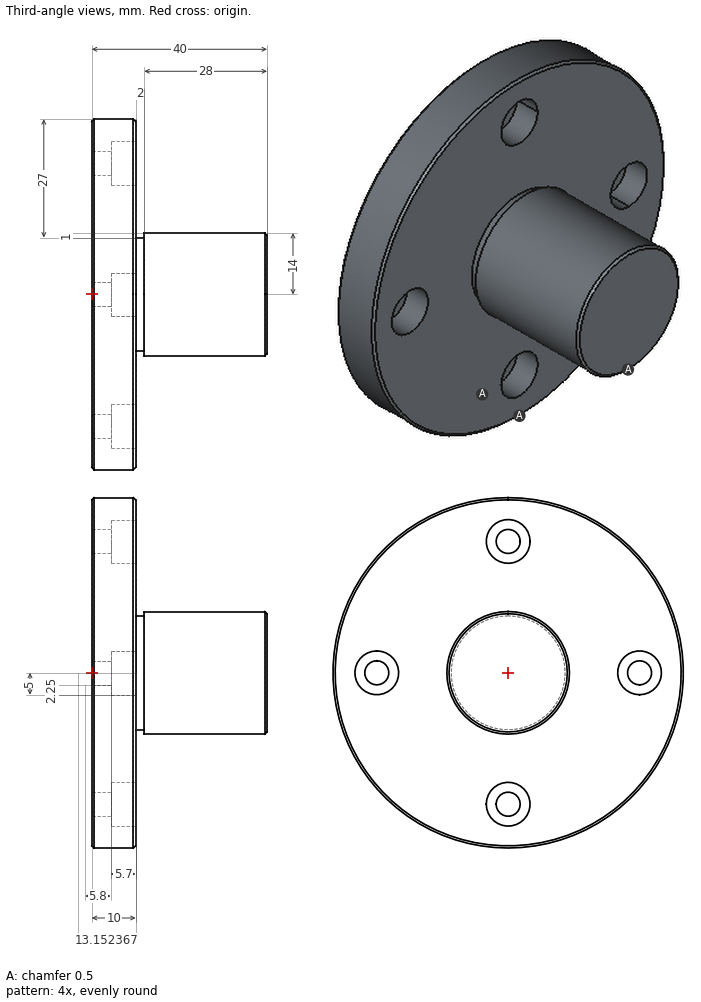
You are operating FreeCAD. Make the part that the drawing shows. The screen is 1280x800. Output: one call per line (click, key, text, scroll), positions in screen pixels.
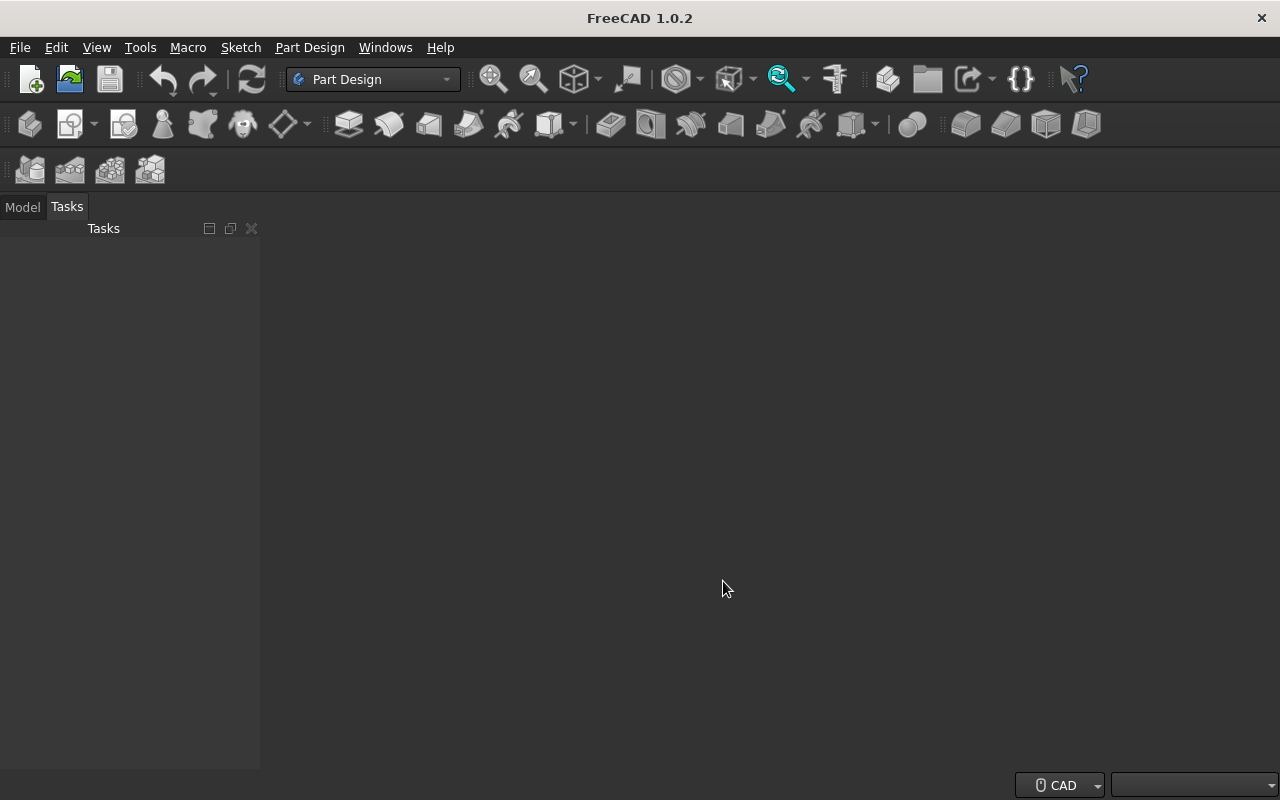
click(30, 80)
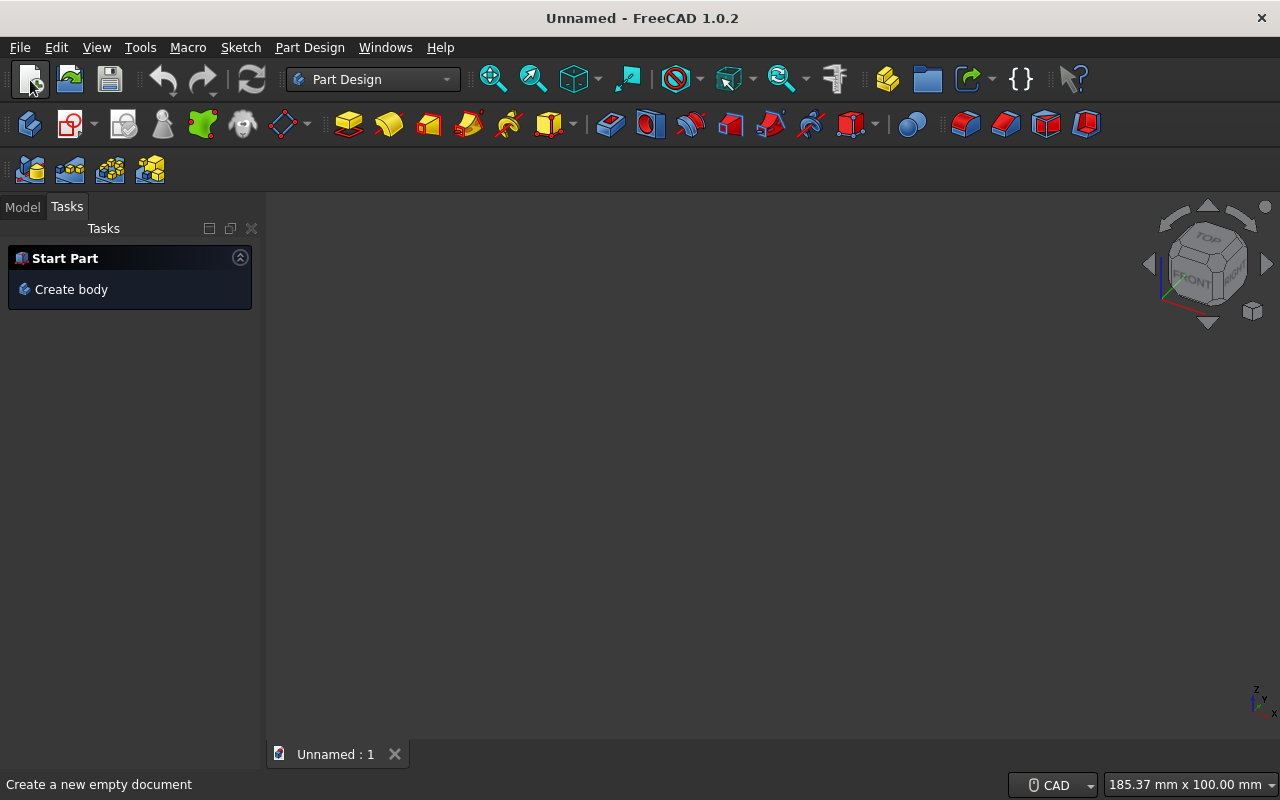
click(70, 124)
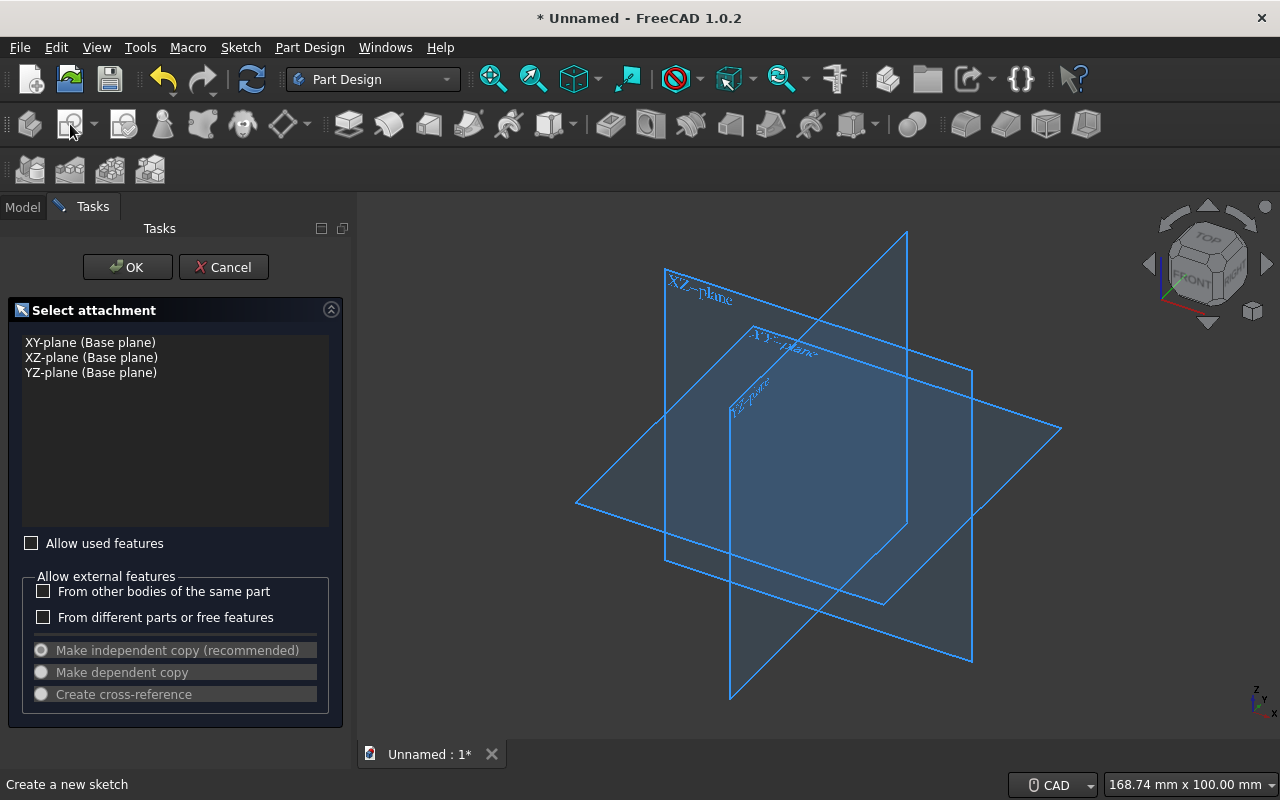
click(82, 342)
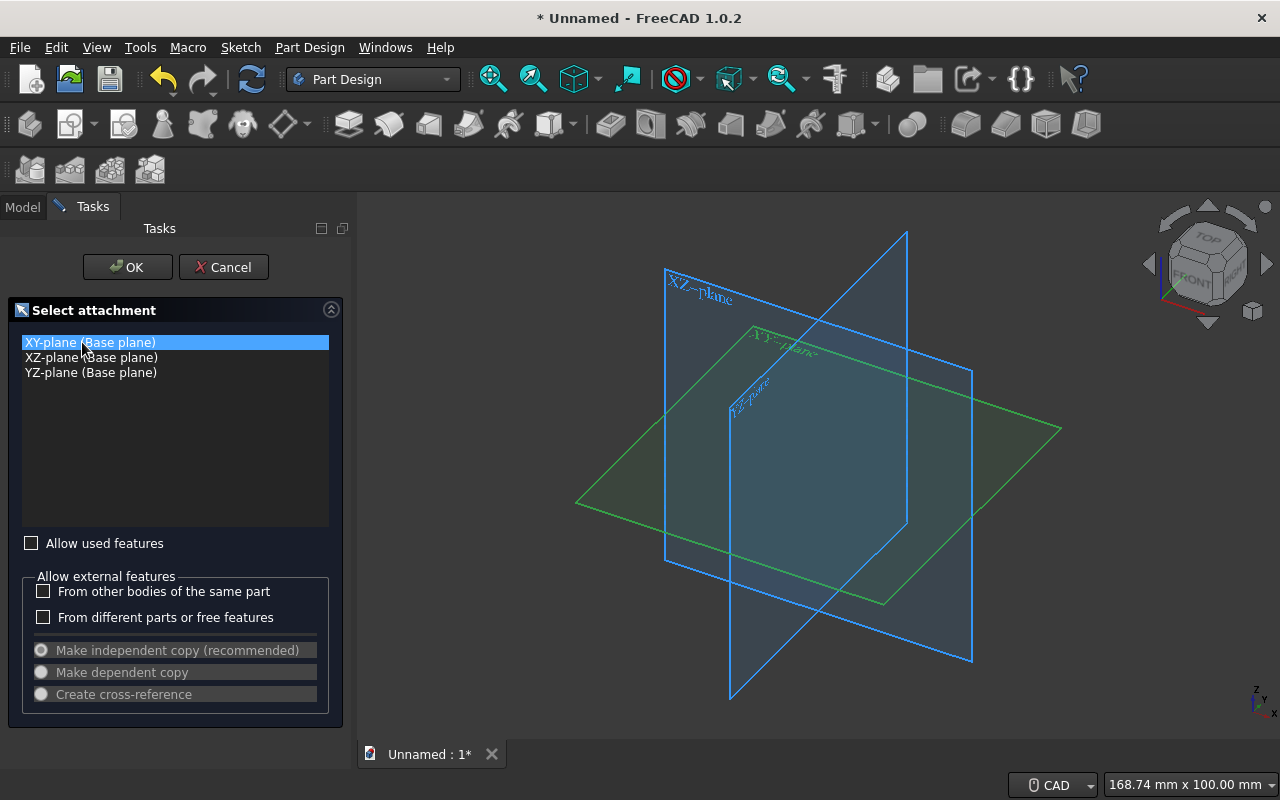
click(128, 267)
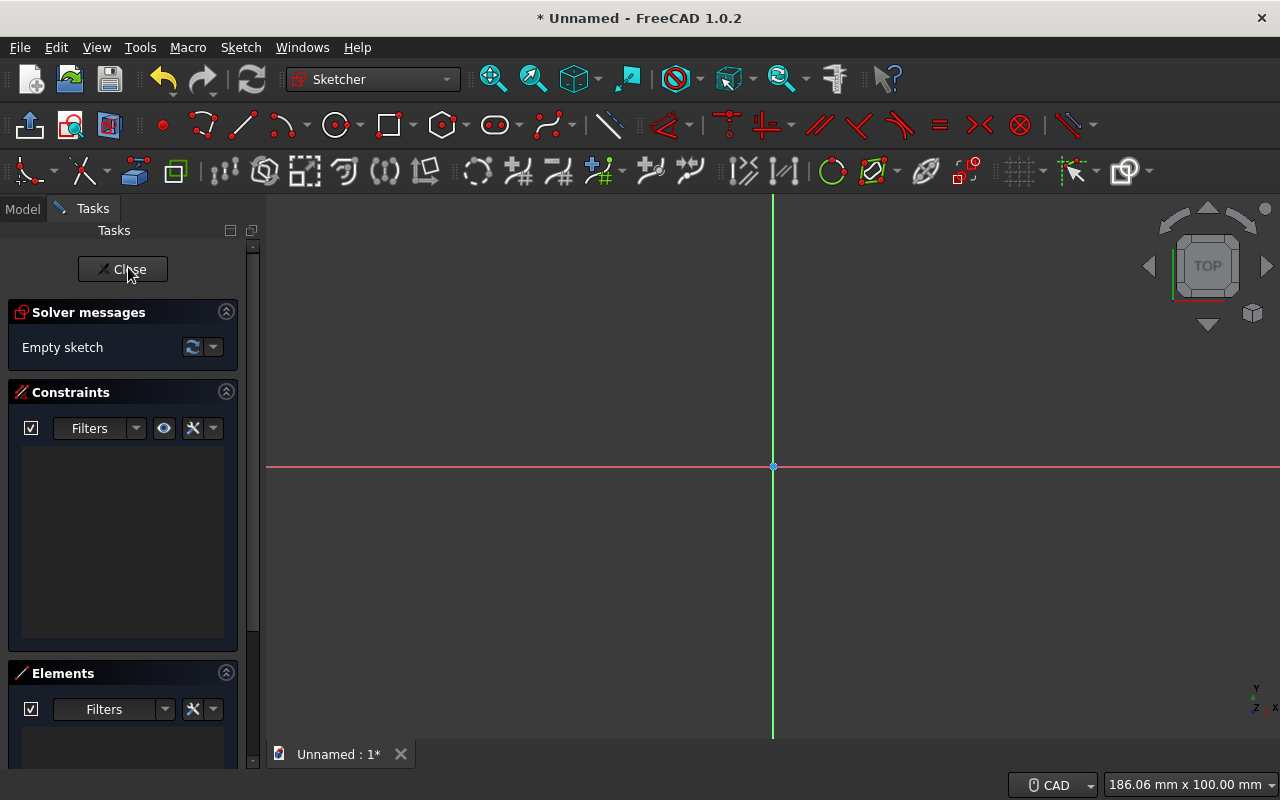
scroll(1115, 222, up, 2)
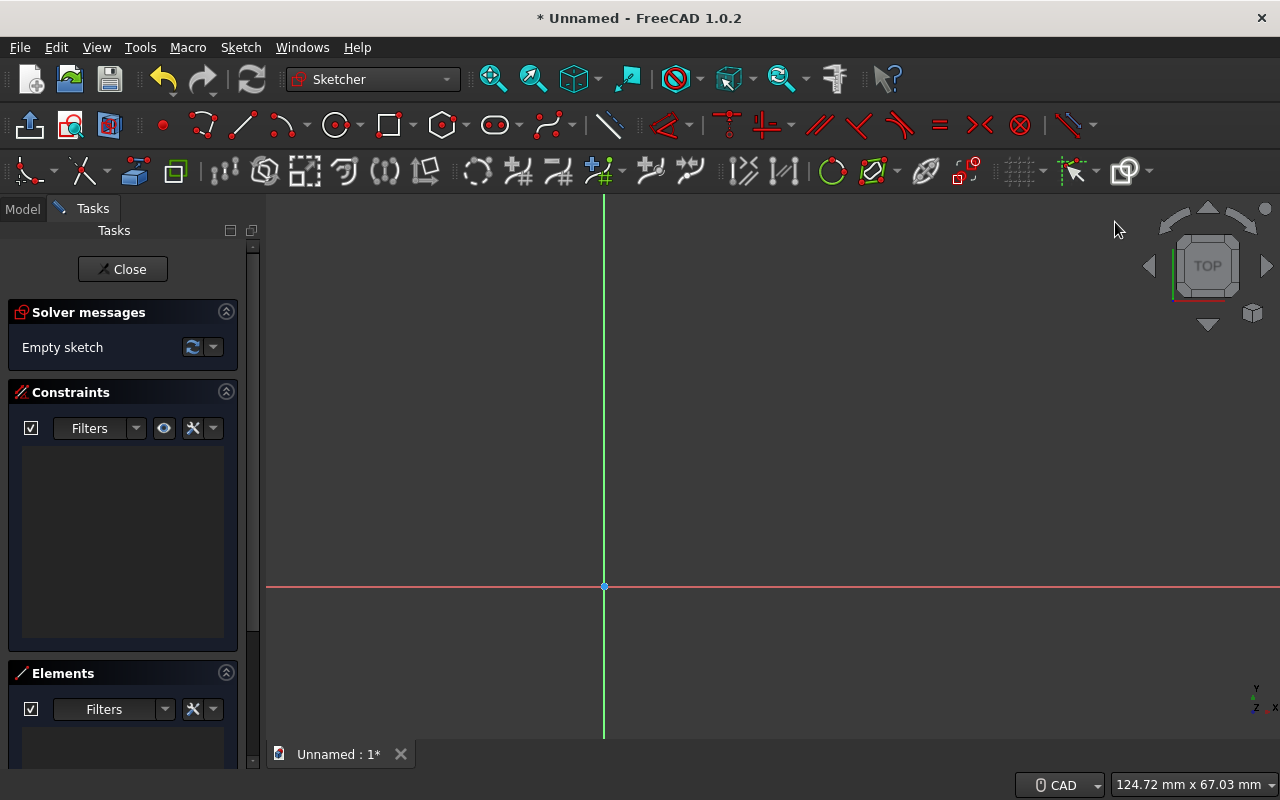
click(204, 126)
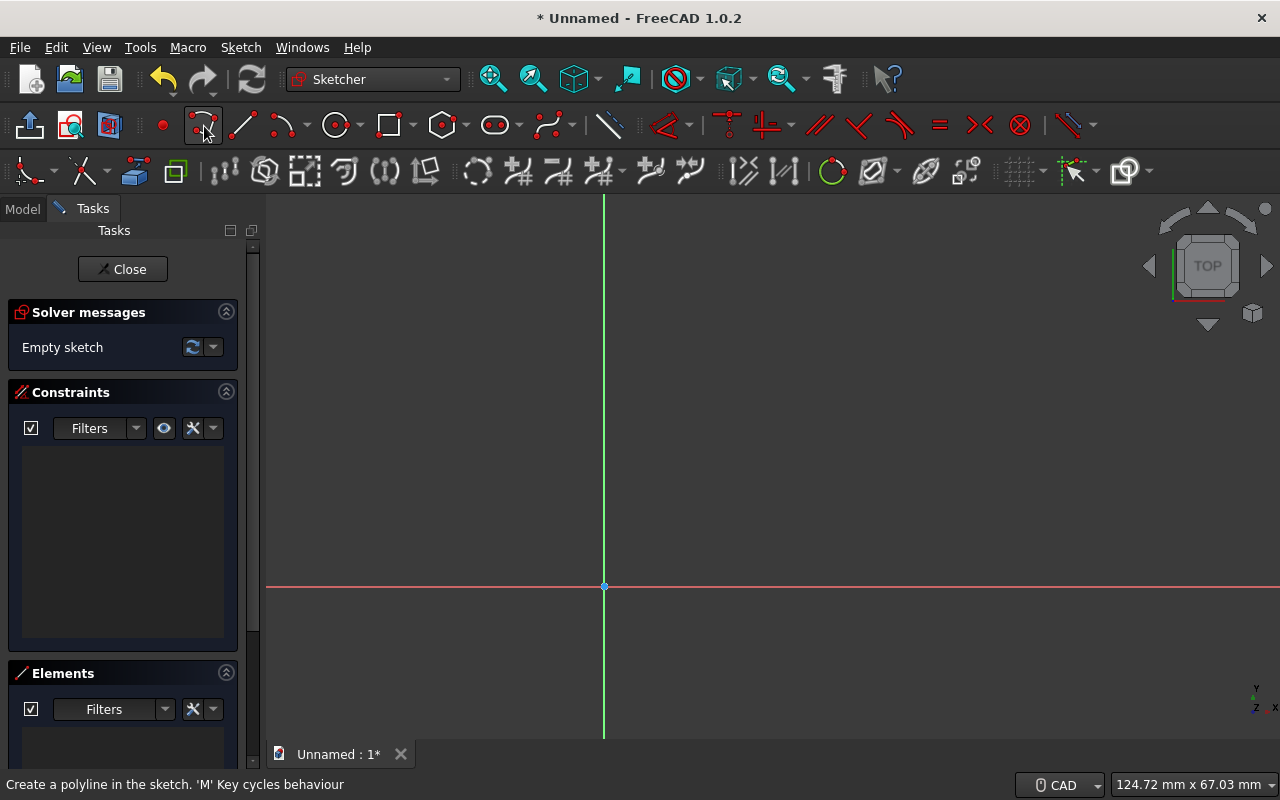
click(604, 587)
click(930, 578)
click(930, 473)
click(702, 473)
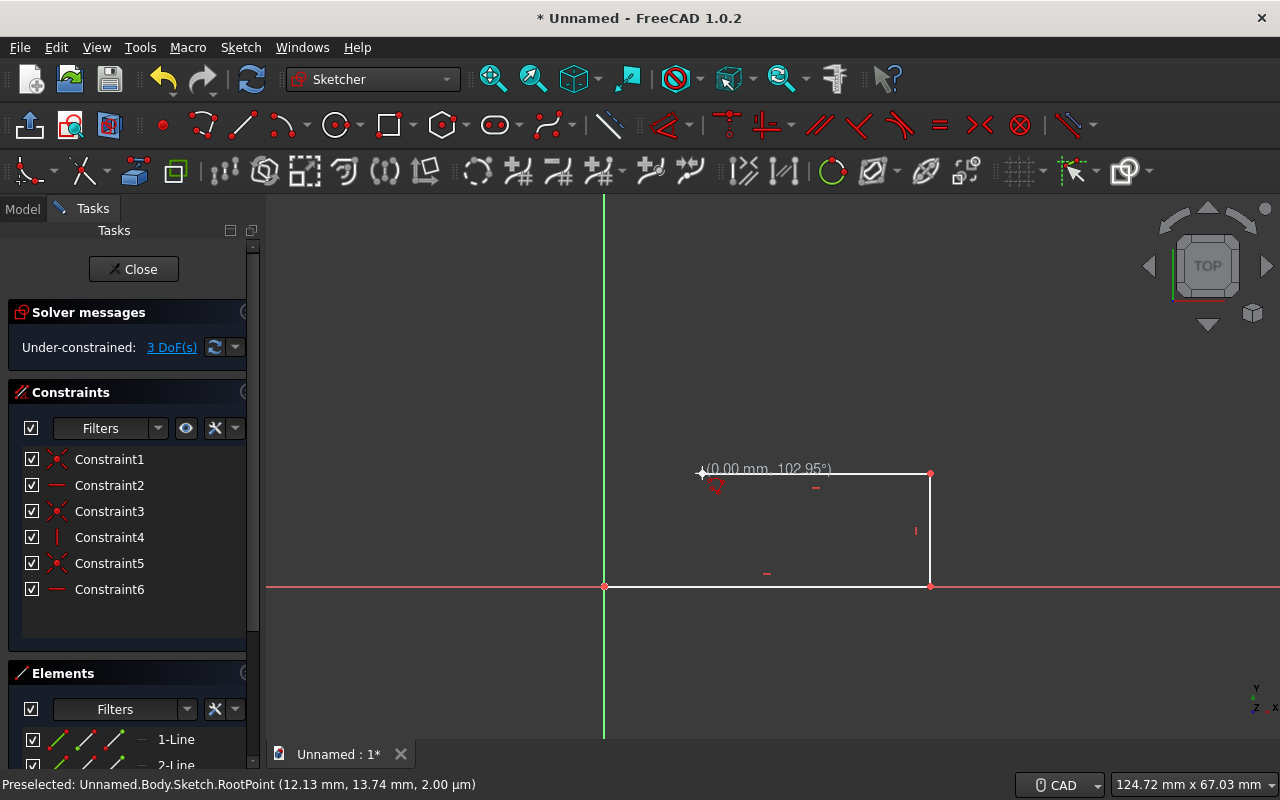
scroll(702, 481, up, 4)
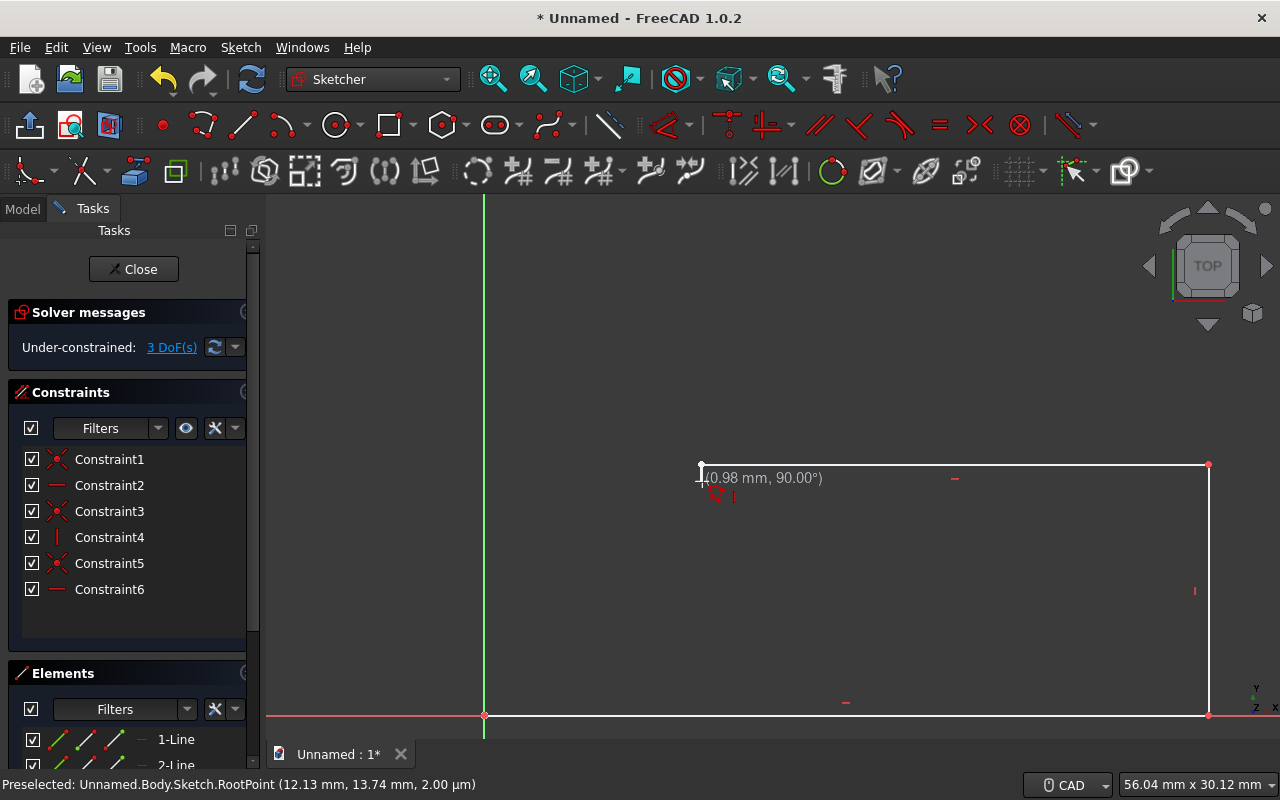
click(701, 480)
click(665, 480)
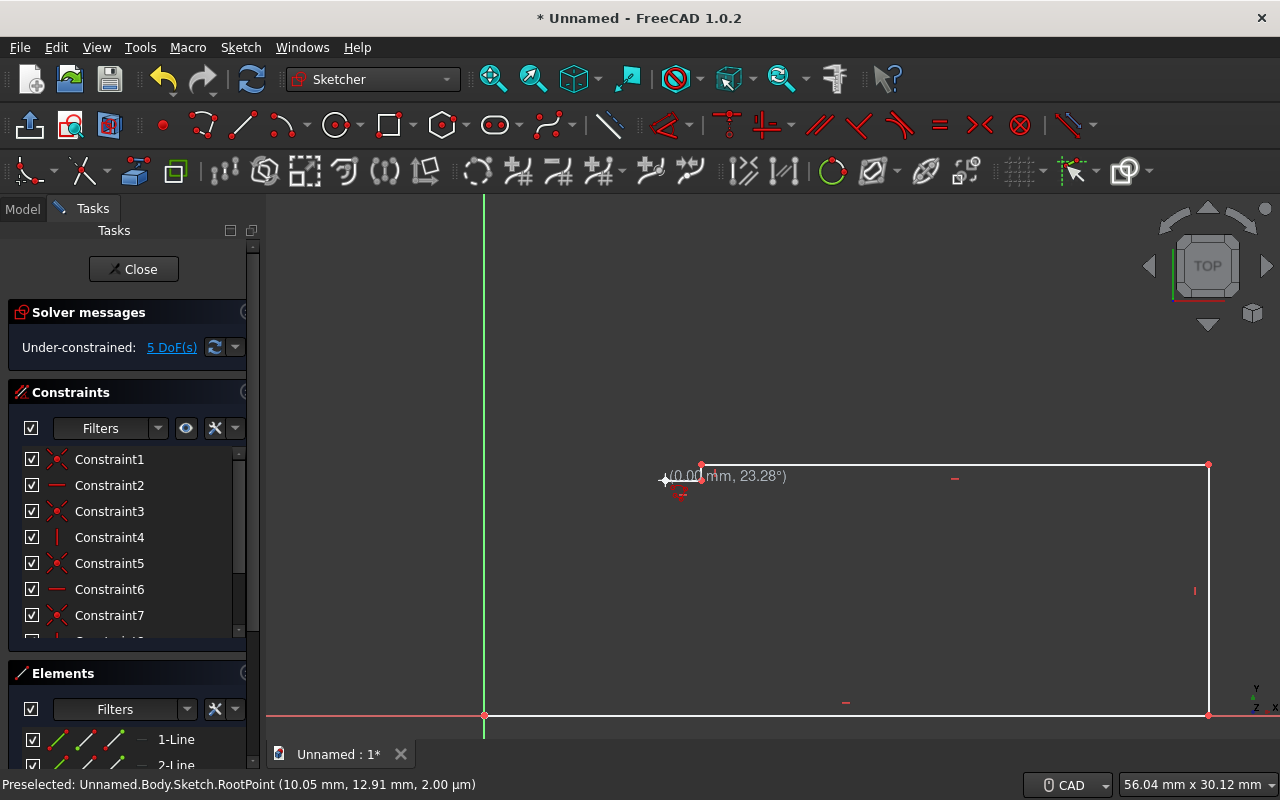
scroll(589, 558, down, 4)